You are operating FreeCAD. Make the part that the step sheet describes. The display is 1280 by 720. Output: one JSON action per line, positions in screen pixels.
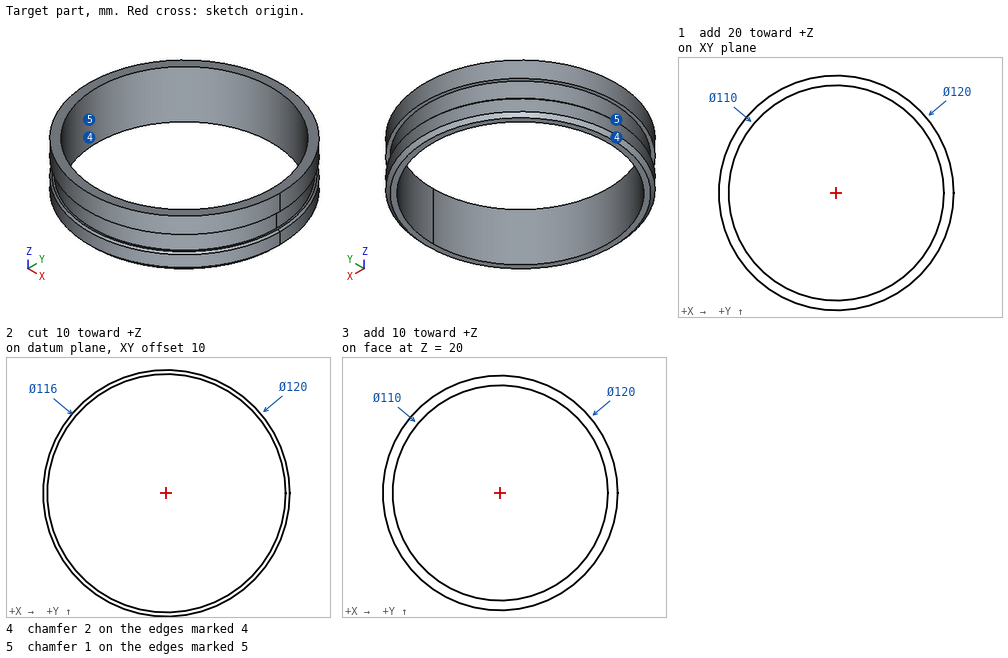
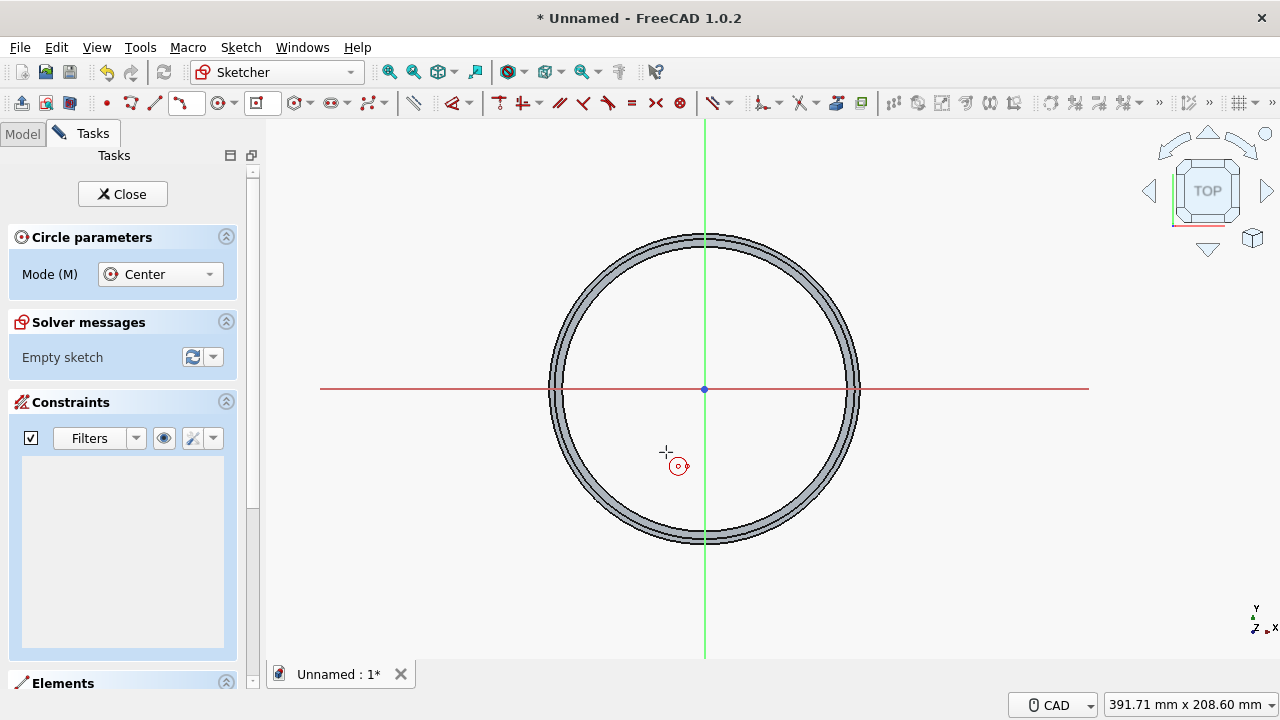
{"action": "left_click", "coordinate": [705, 389]}
{"action": "left_click", "coordinate": [814, 279]}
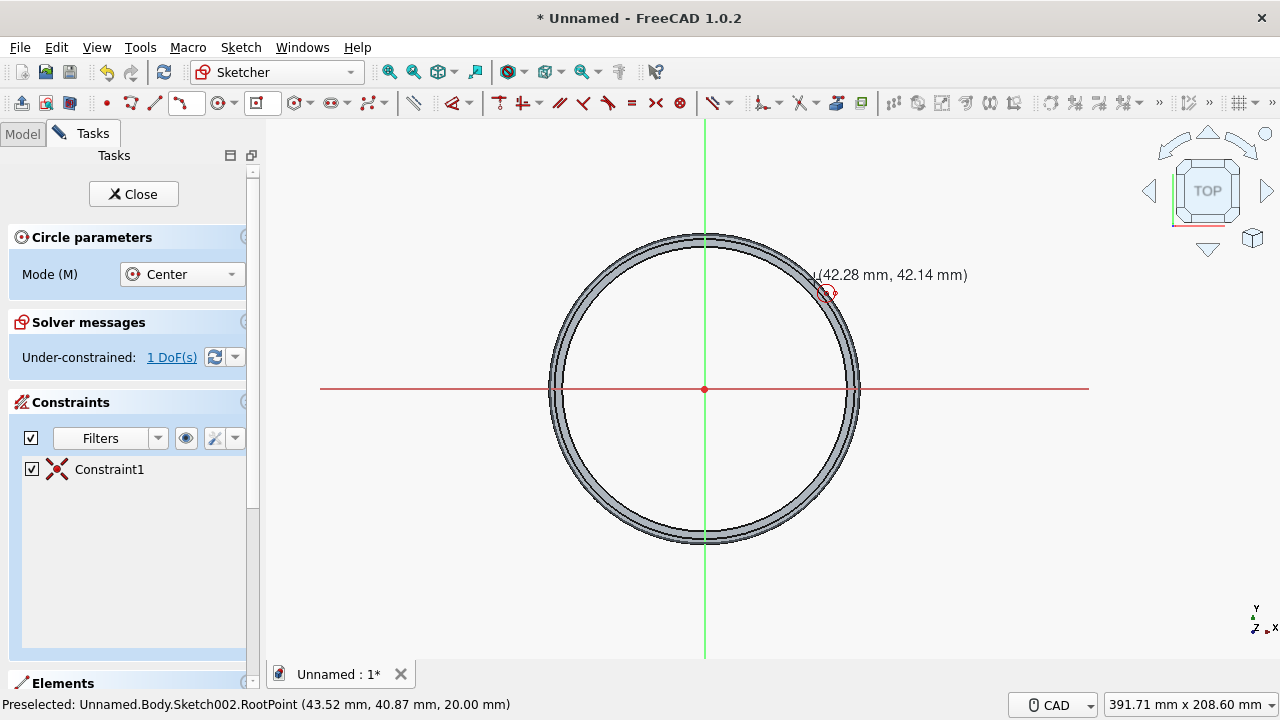
{"action": "left_click", "coordinate": [705, 389]}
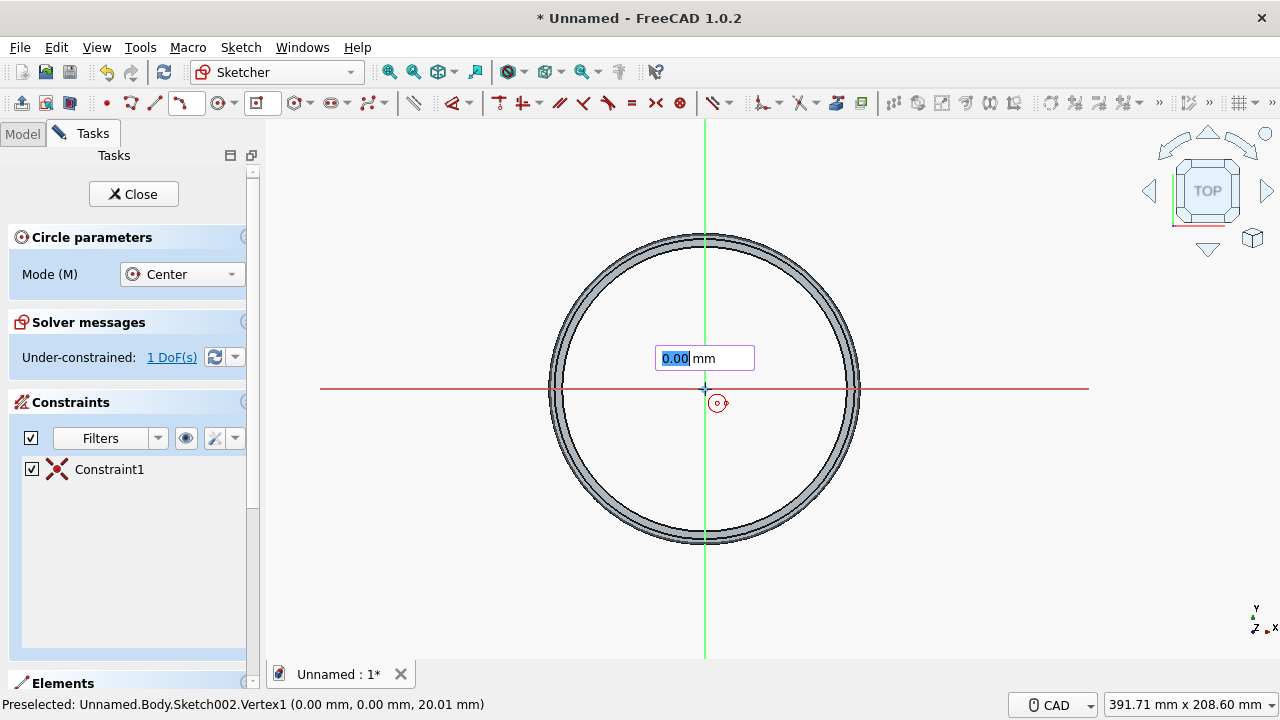
{"action": "scroll", "coordinate": [805, 288], "scroll_direction": "up", "scroll_amount": 2}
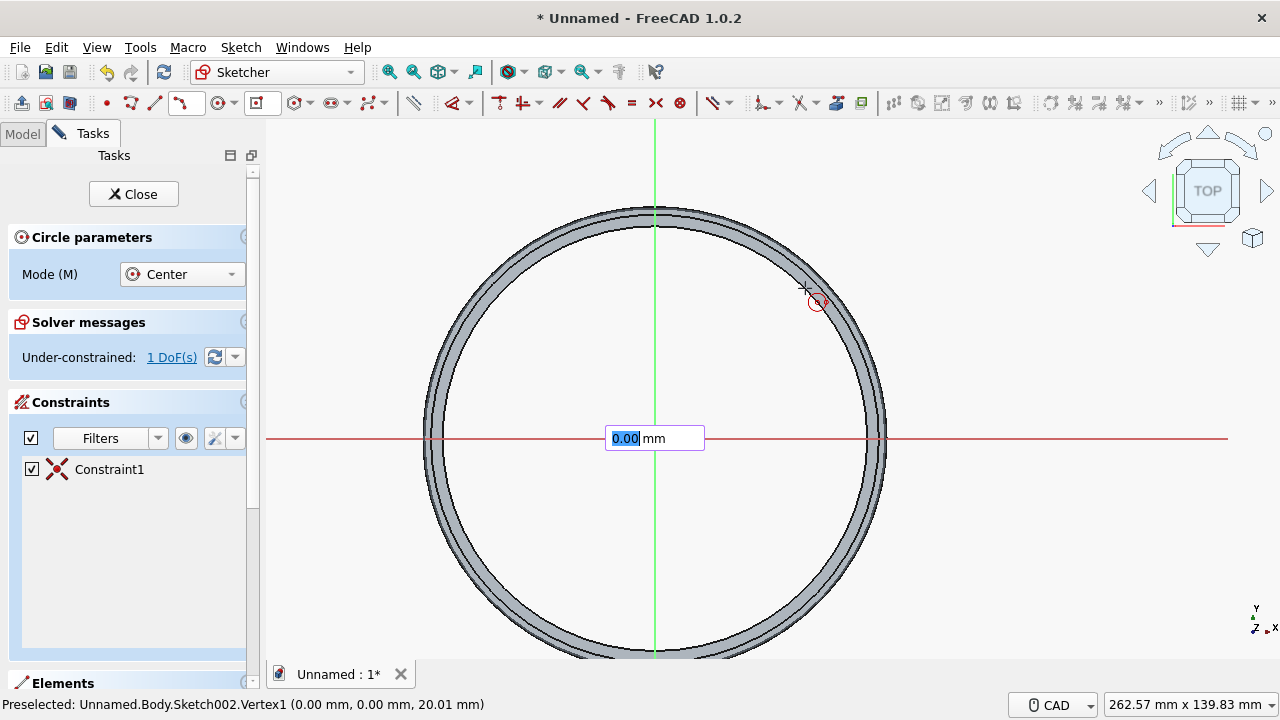
{"action": "left_click", "coordinate": [805, 288]}
{"action": "key", "text": "Escape"}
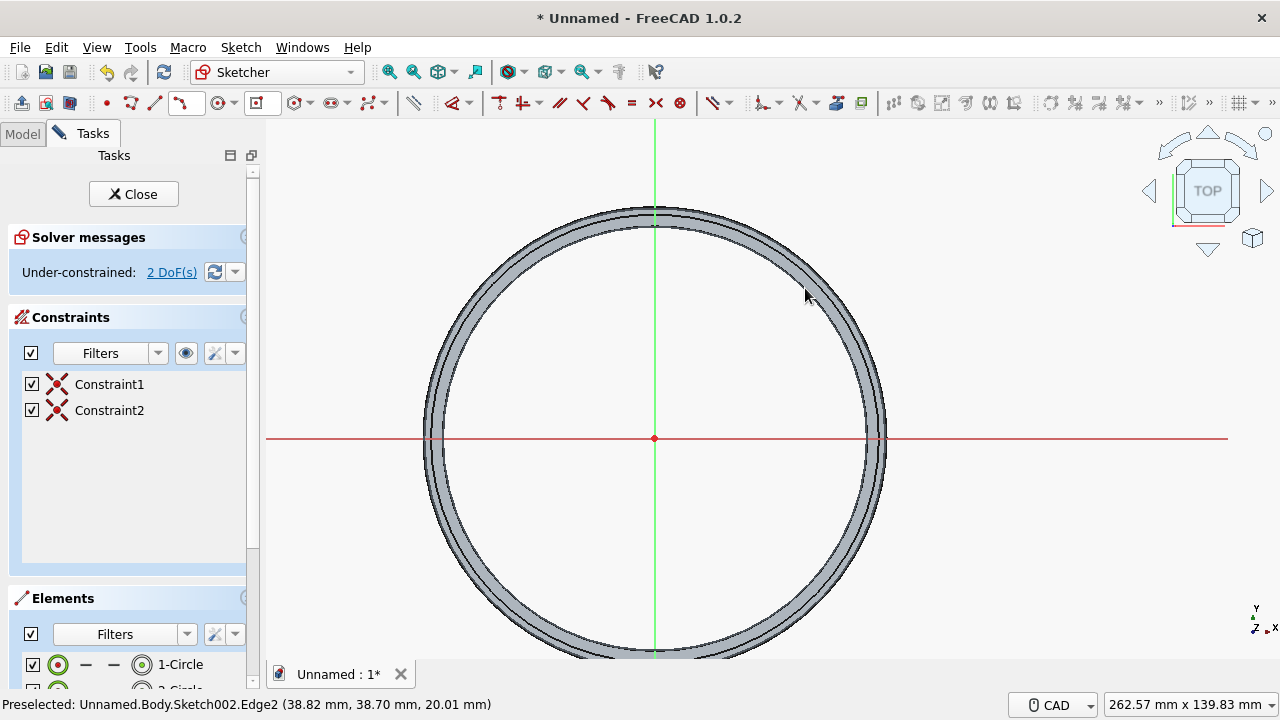
{"action": "left_click", "coordinate": [817, 275]}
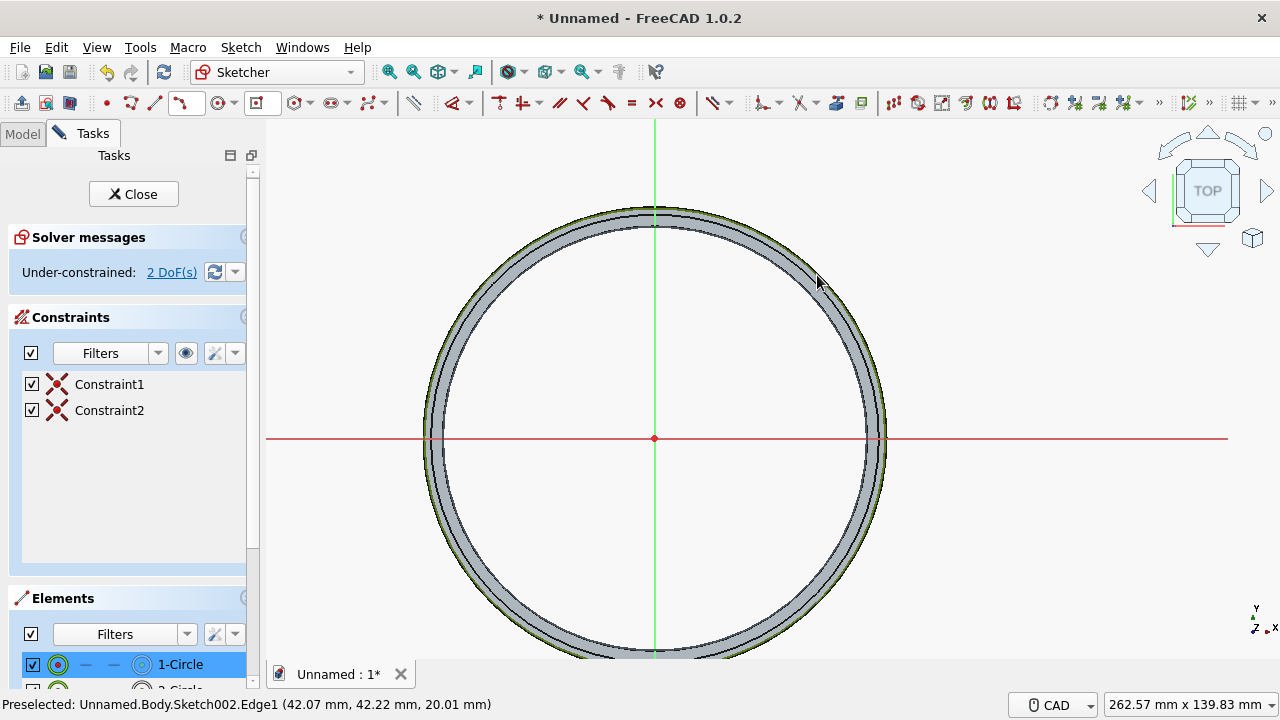
{"action": "left_click", "coordinate": [472, 104]}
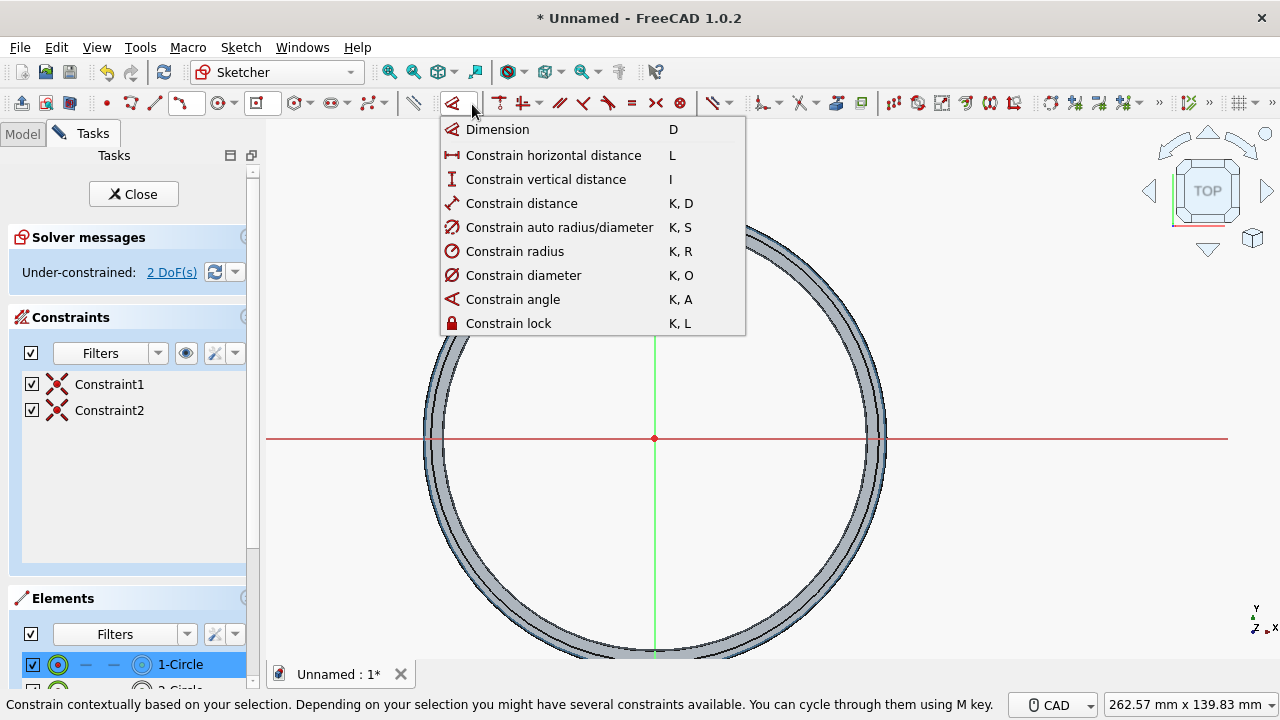
{"action": "left_click", "coordinate": [593, 275]}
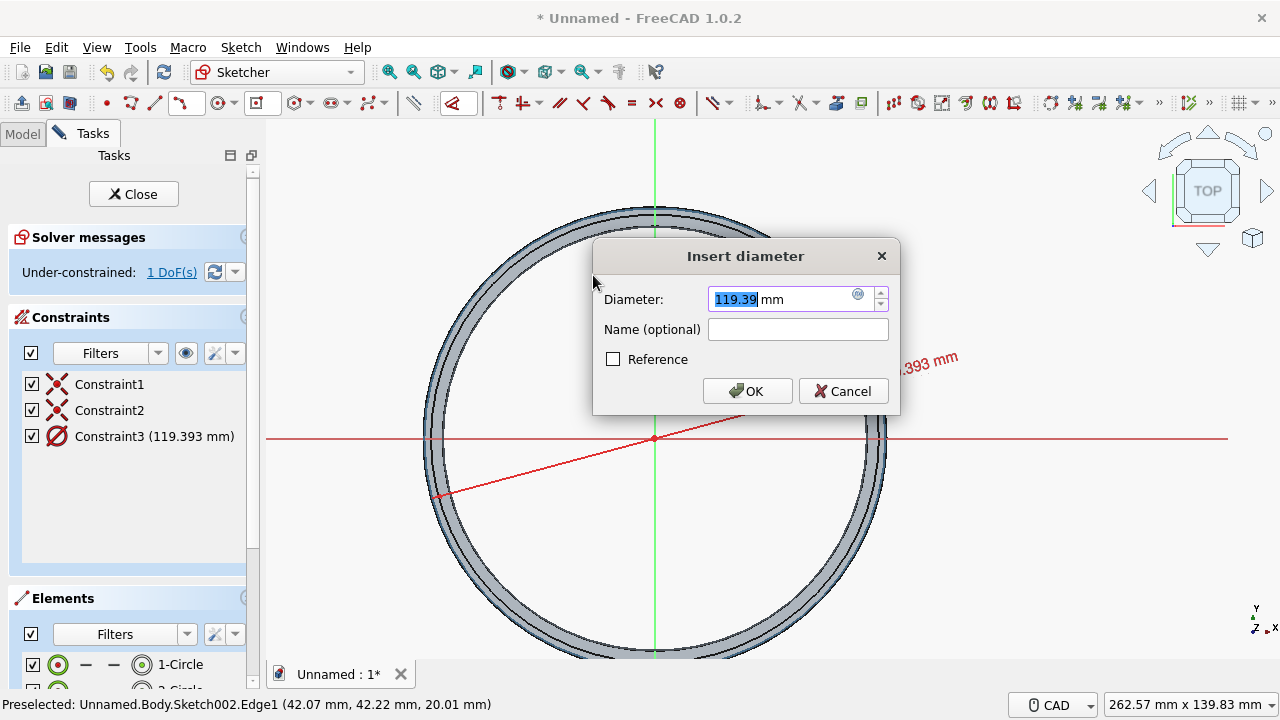
{"action": "type", "text": "120"}
{"action": "key", "text": "Return"}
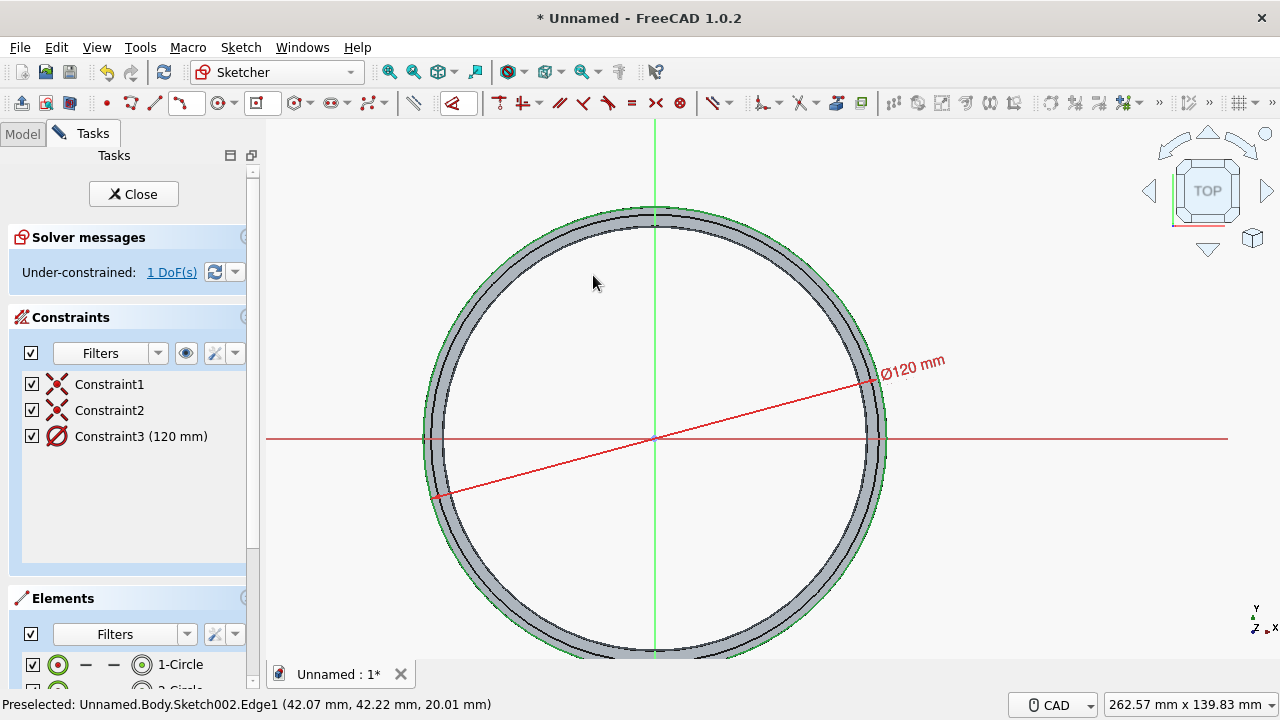
{"action": "left_click", "coordinate": [804, 288]}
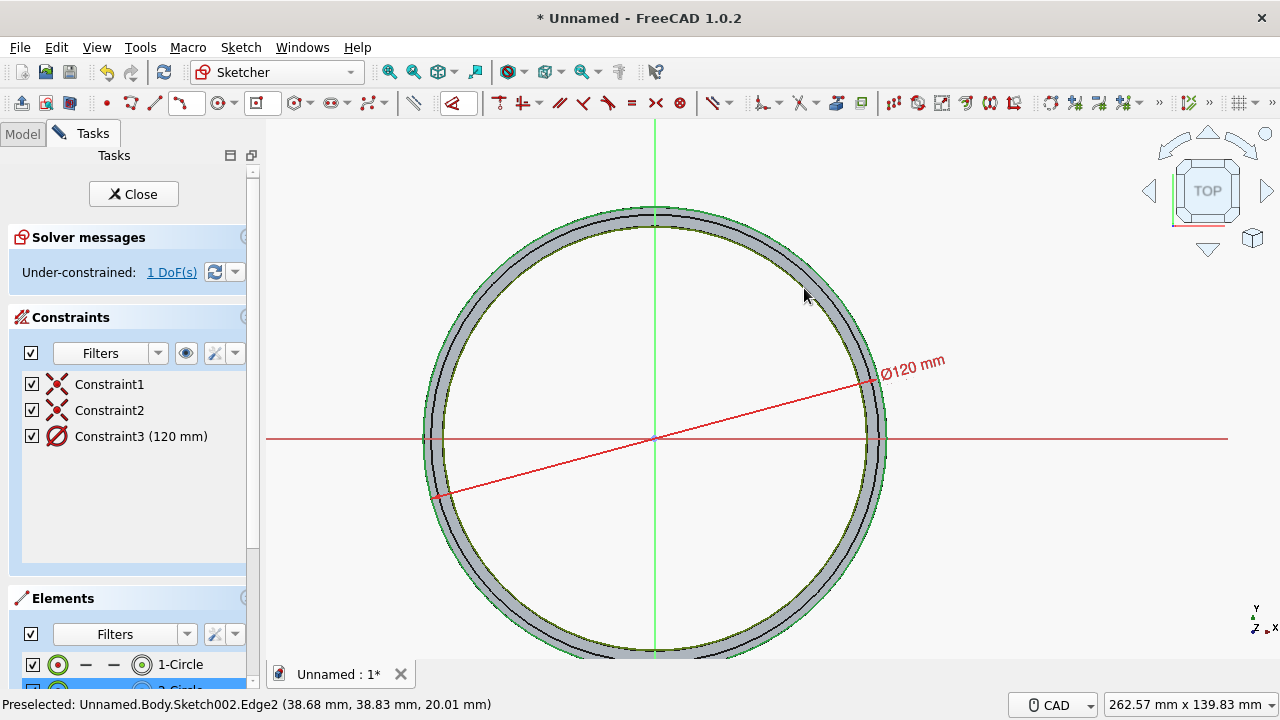
{"action": "key", "text": "k o"}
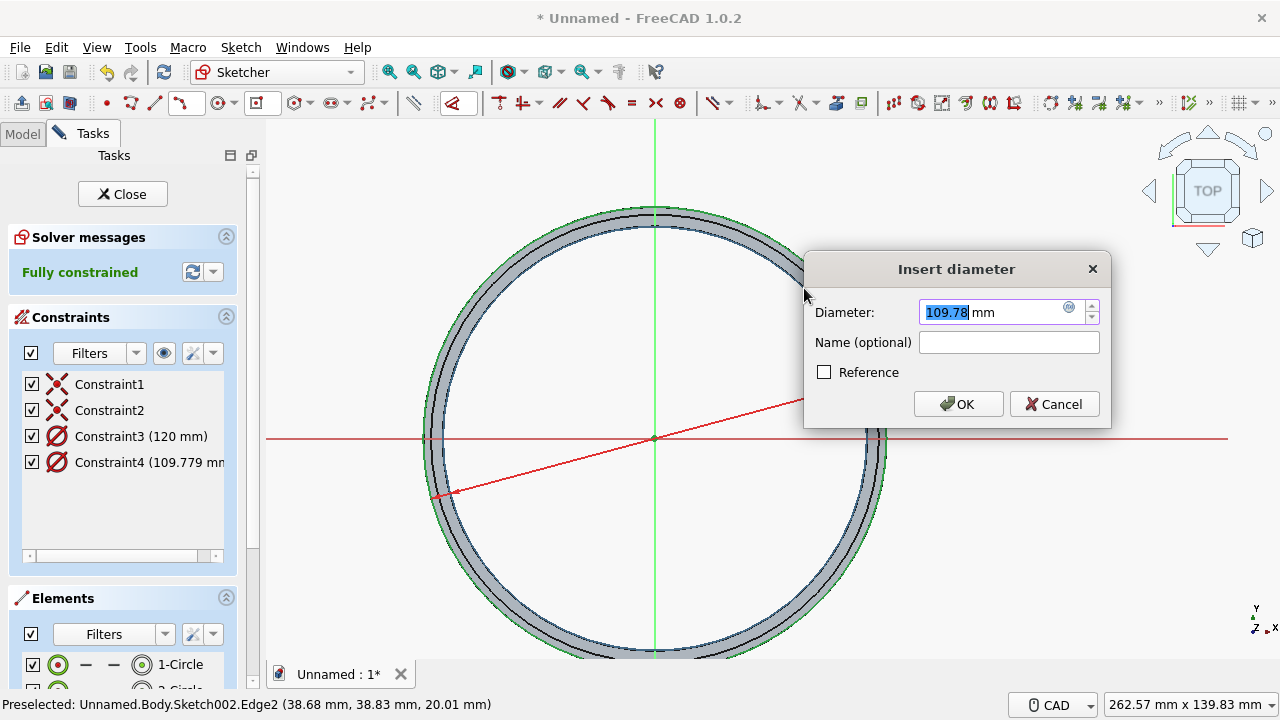
{"action": "type", "text": "110"}
{"action": "key", "text": "Return"}